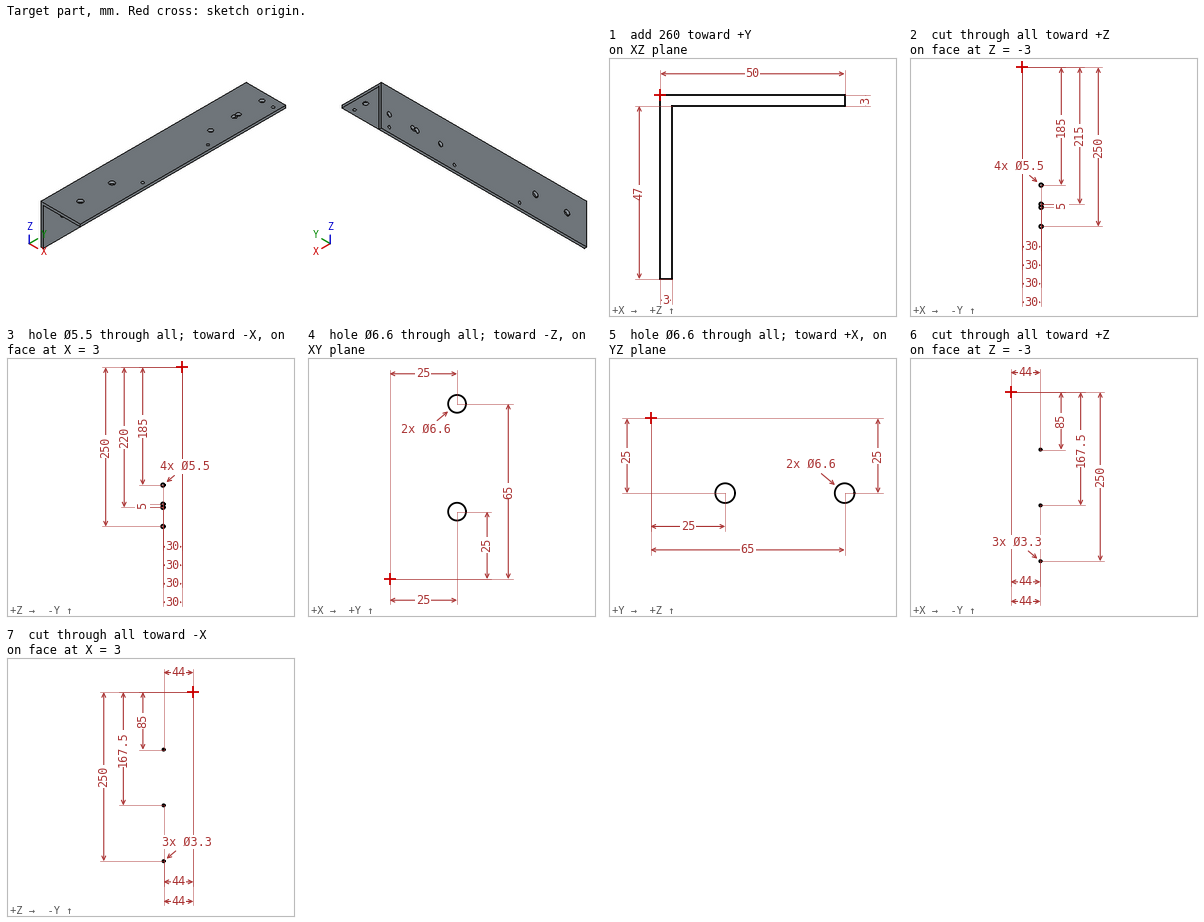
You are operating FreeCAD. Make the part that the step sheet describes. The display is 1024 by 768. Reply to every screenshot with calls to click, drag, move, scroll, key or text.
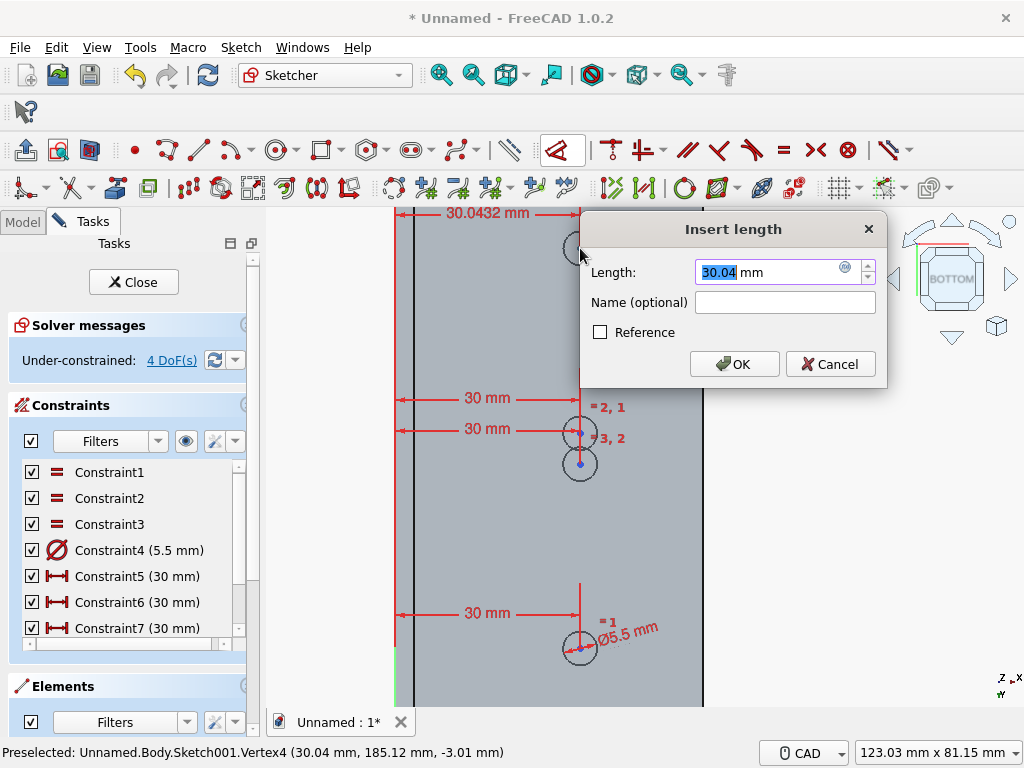
text(30)
key(Return)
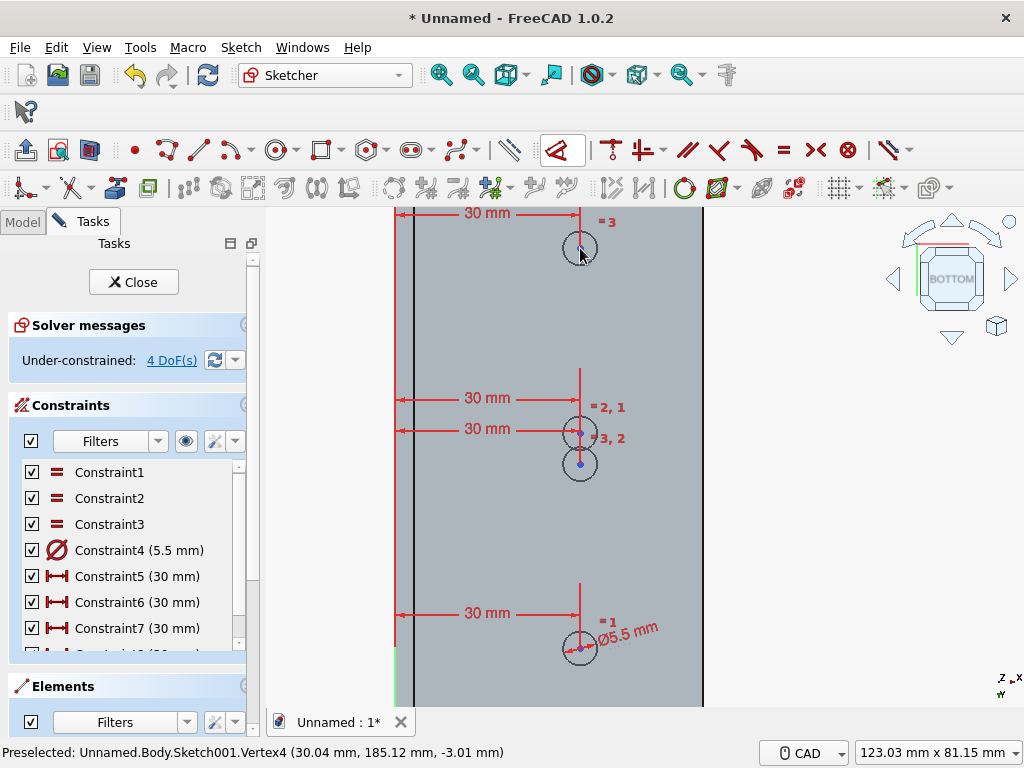
scroll(580, 433, up, 2)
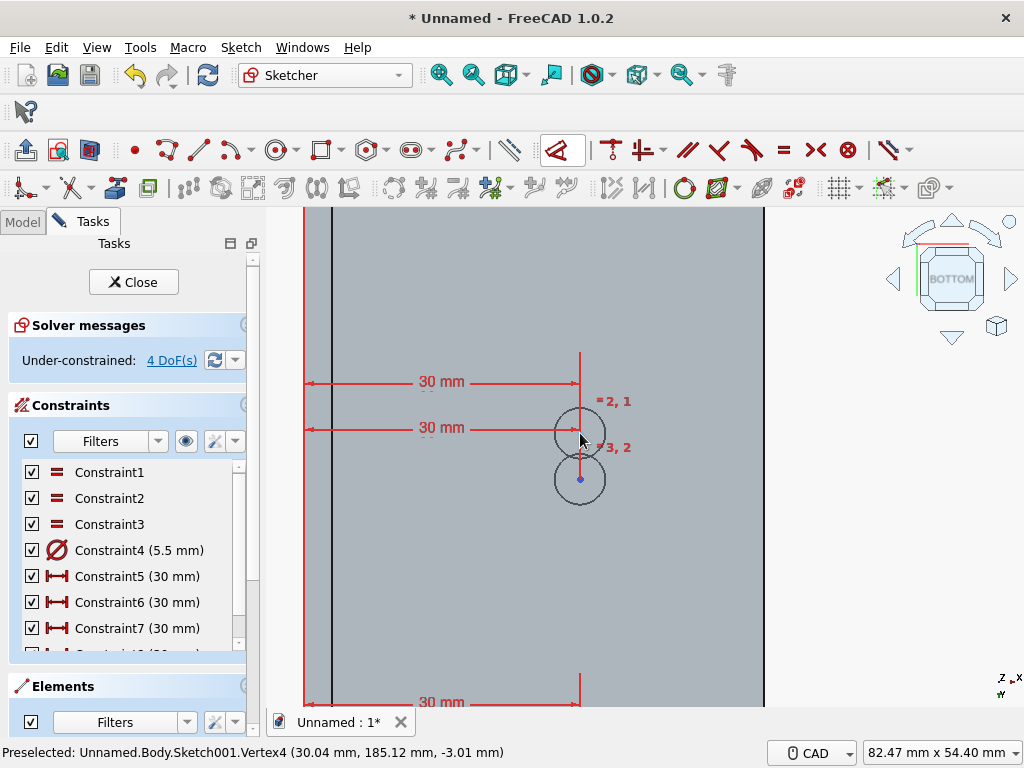
click(580, 433)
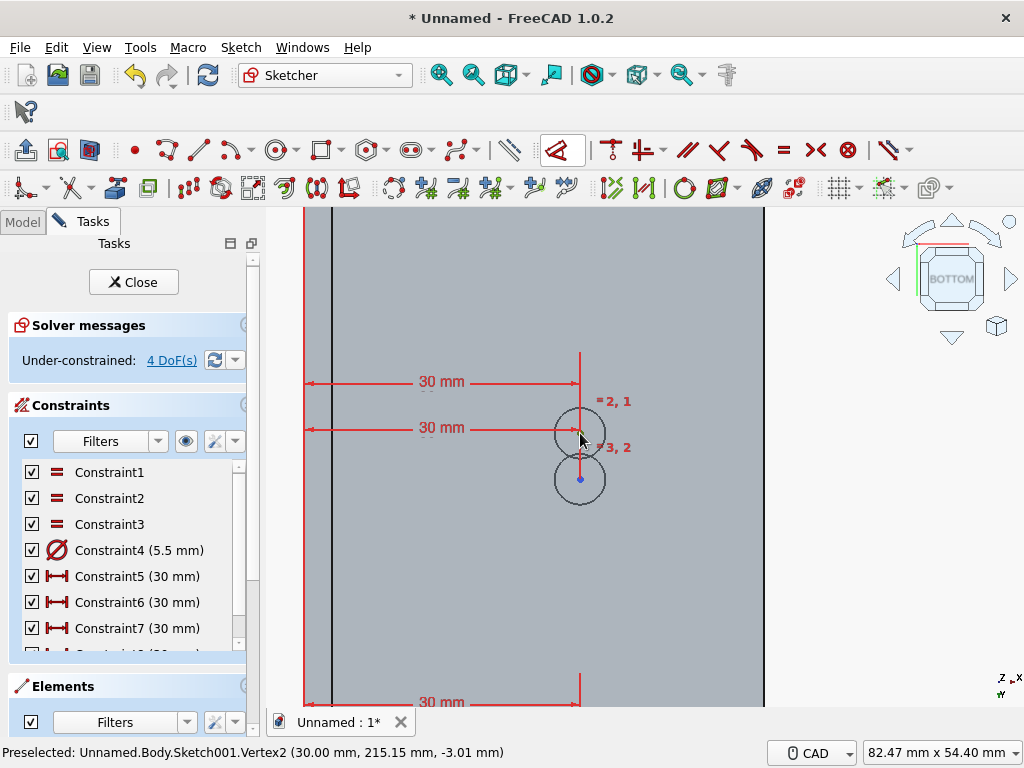
click(580, 479)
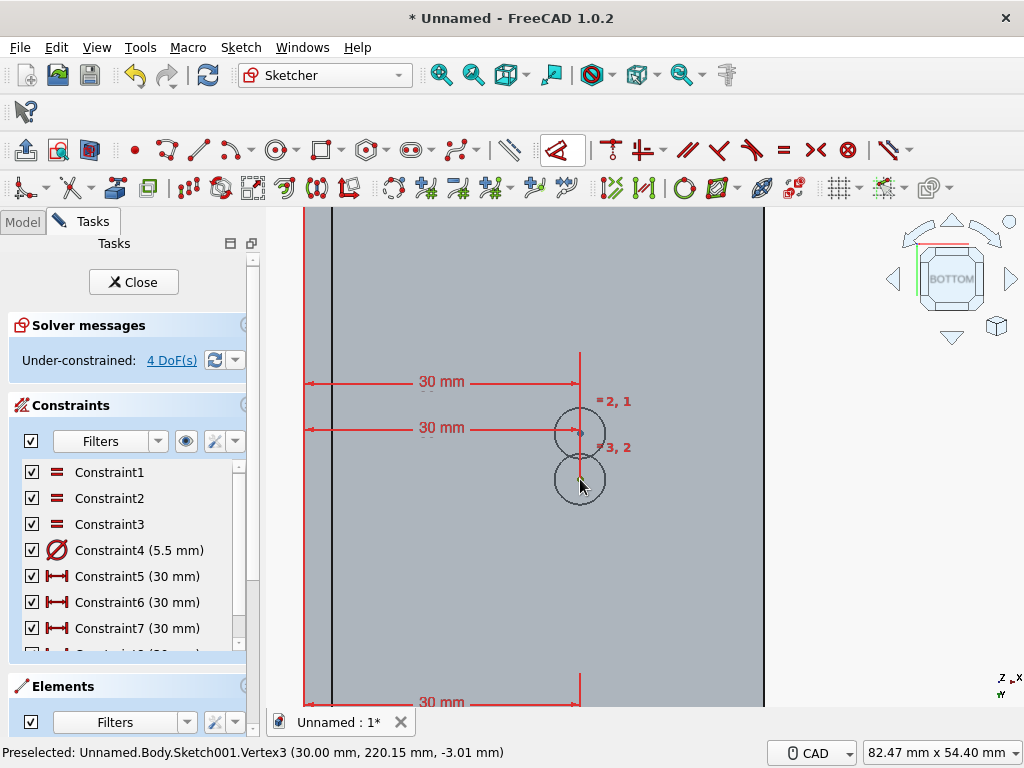
key(i)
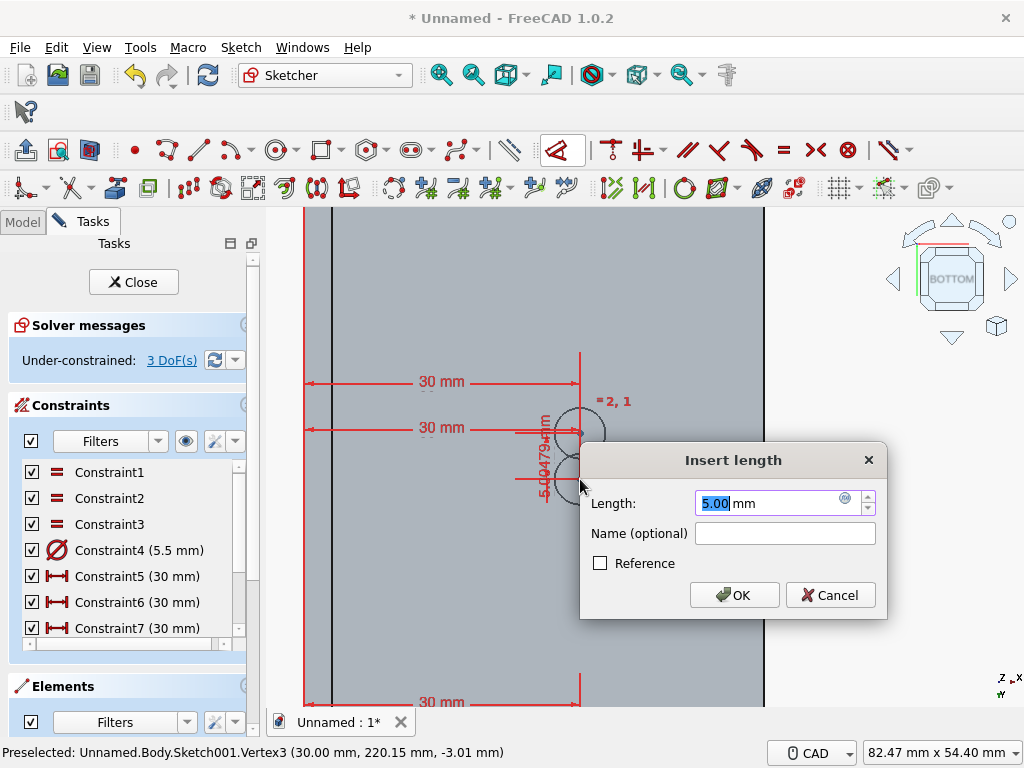
text(5)
key(Return)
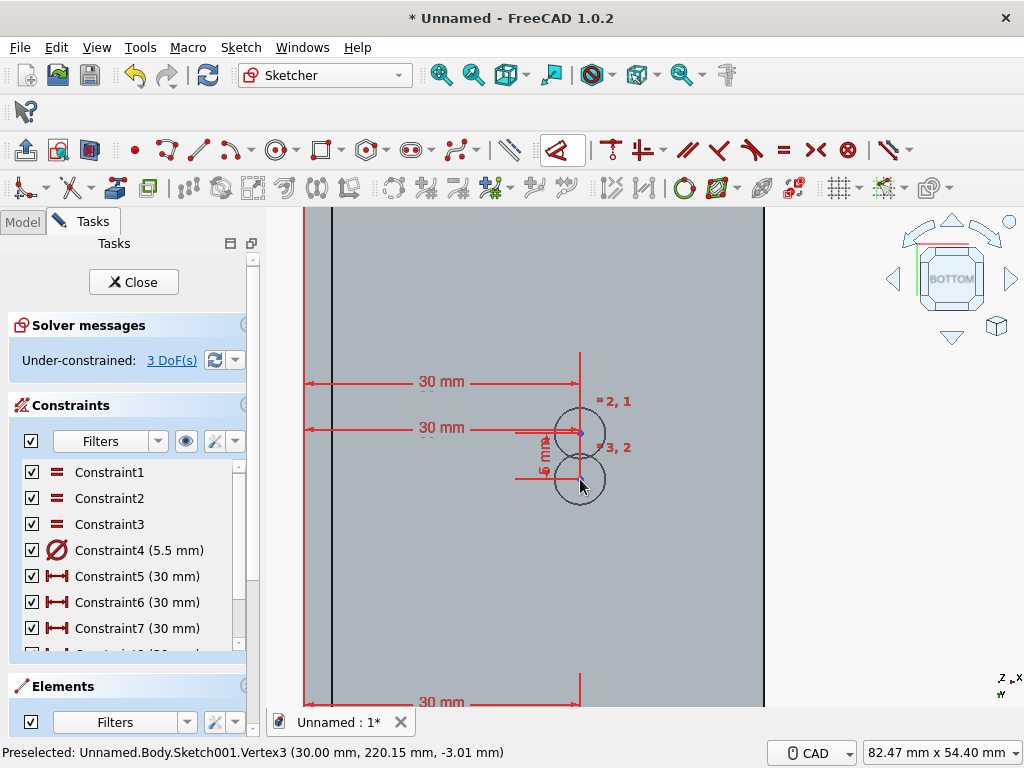
scroll(574, 459, down, 4)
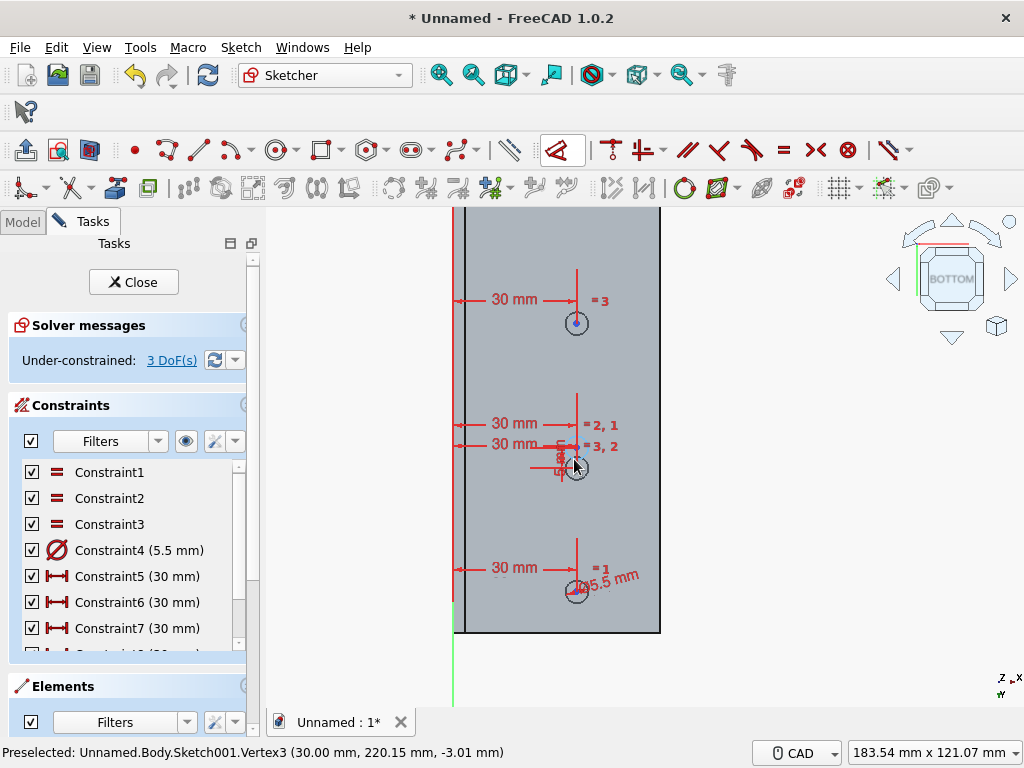
click(577, 592)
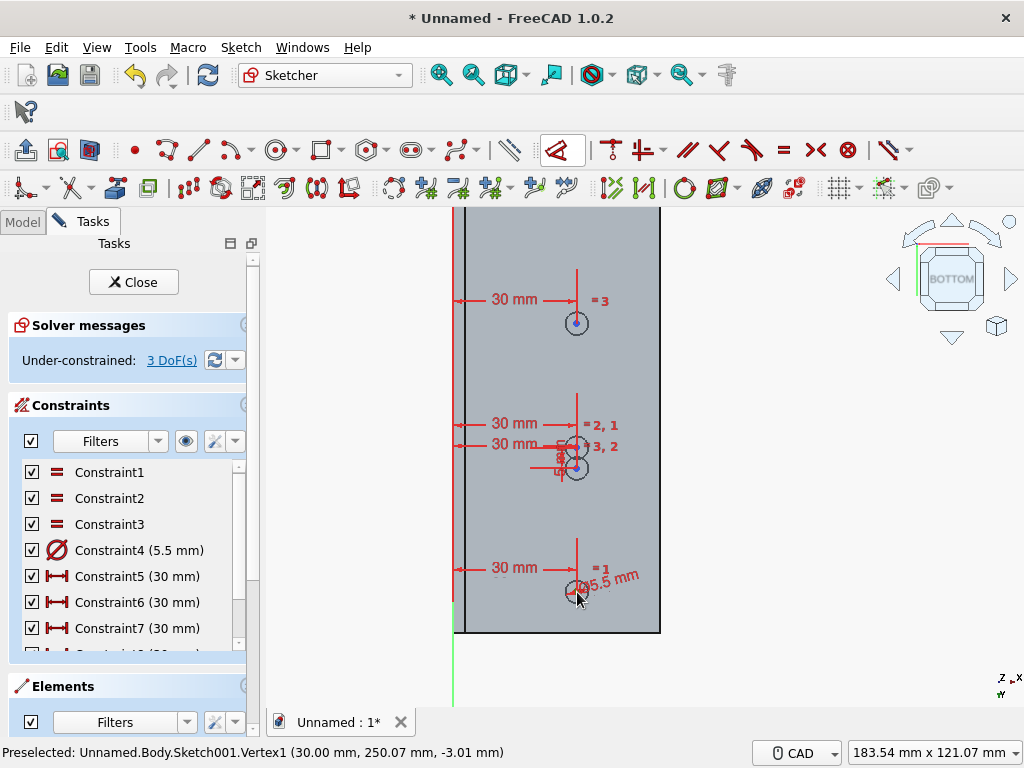
key(i)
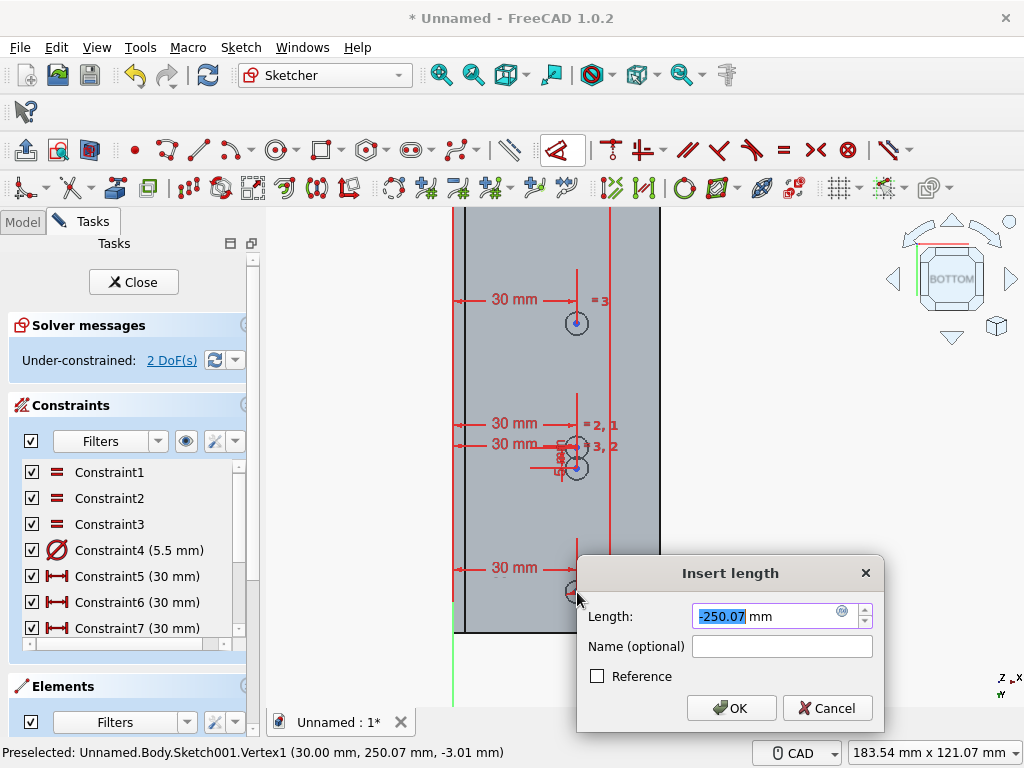
text(-250)
key(Return)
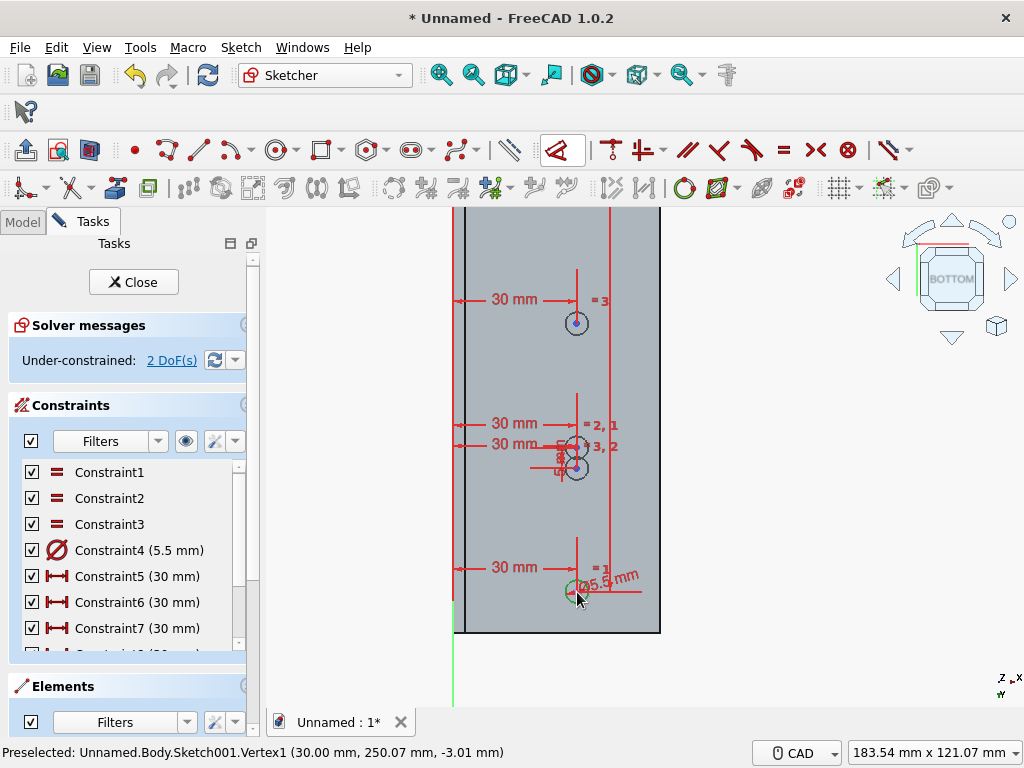
click(577, 448)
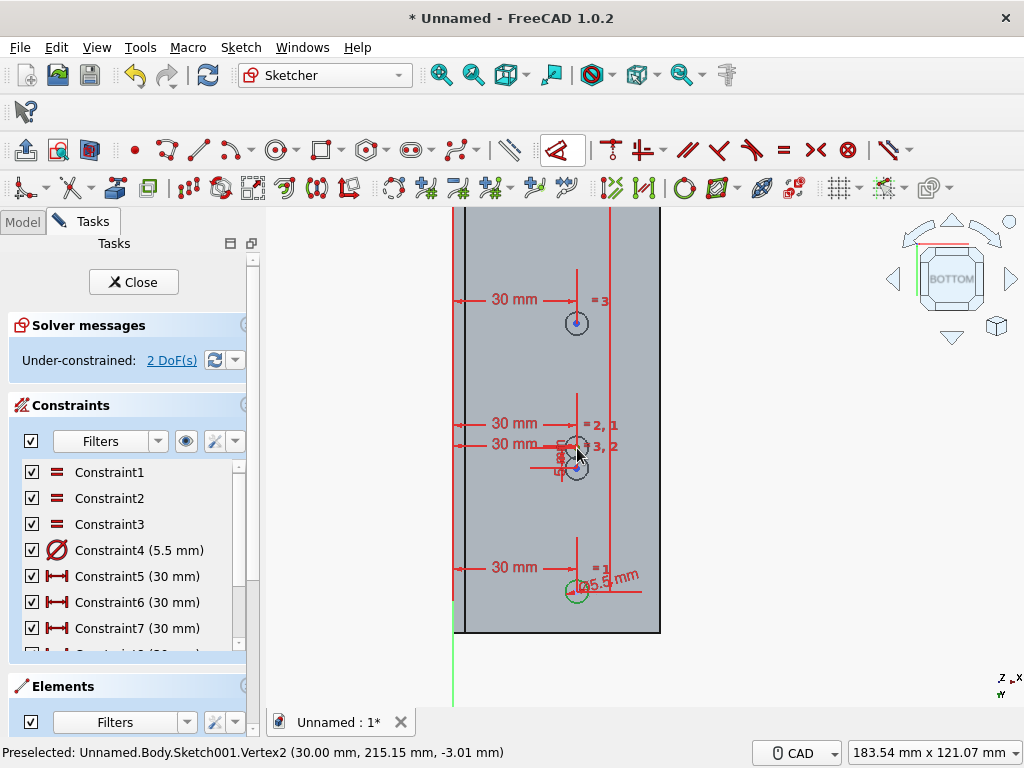
key(i)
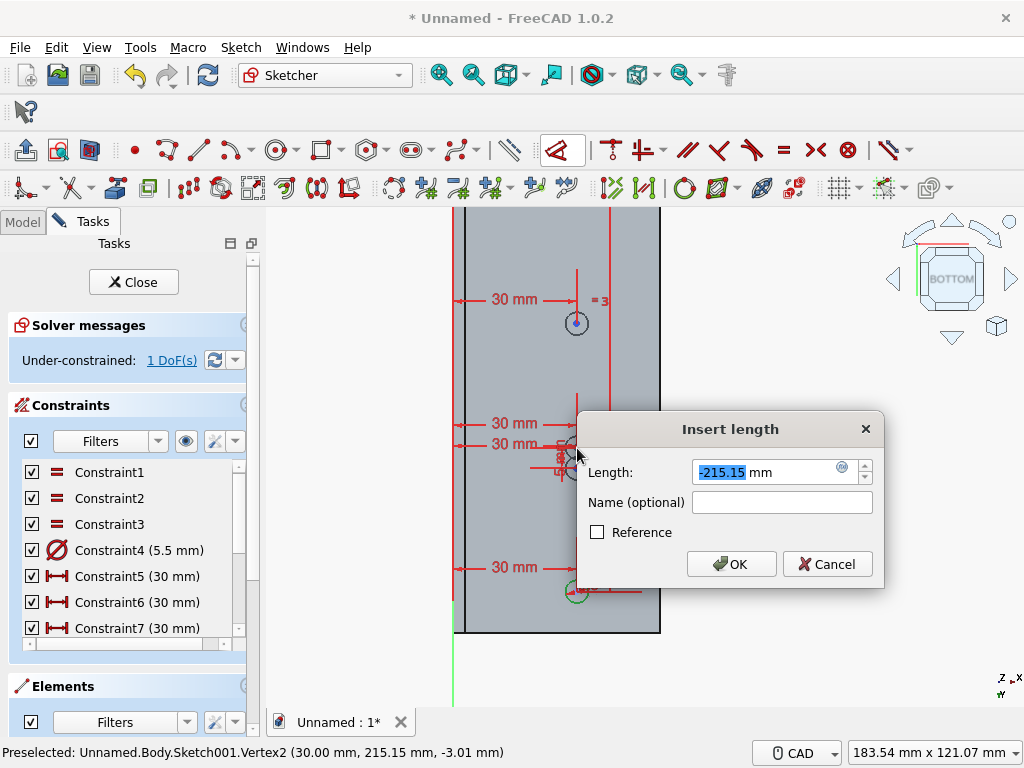
text(-215)
key(Return)